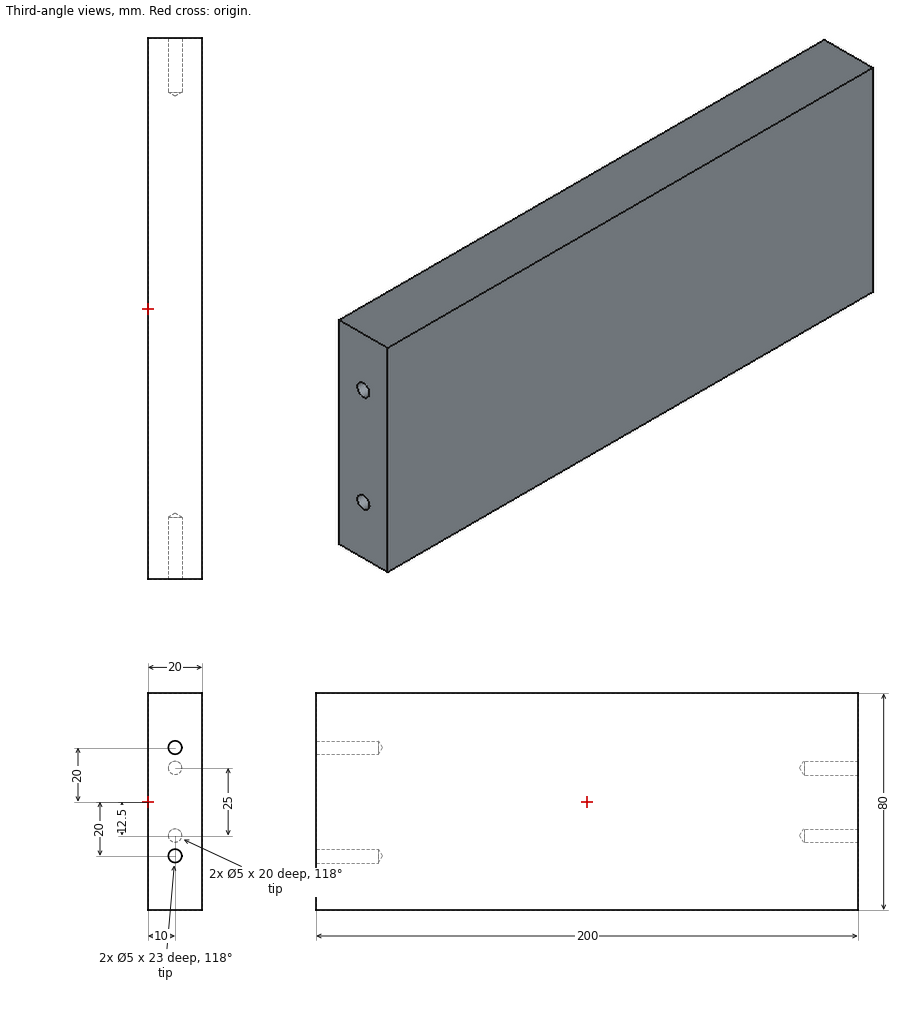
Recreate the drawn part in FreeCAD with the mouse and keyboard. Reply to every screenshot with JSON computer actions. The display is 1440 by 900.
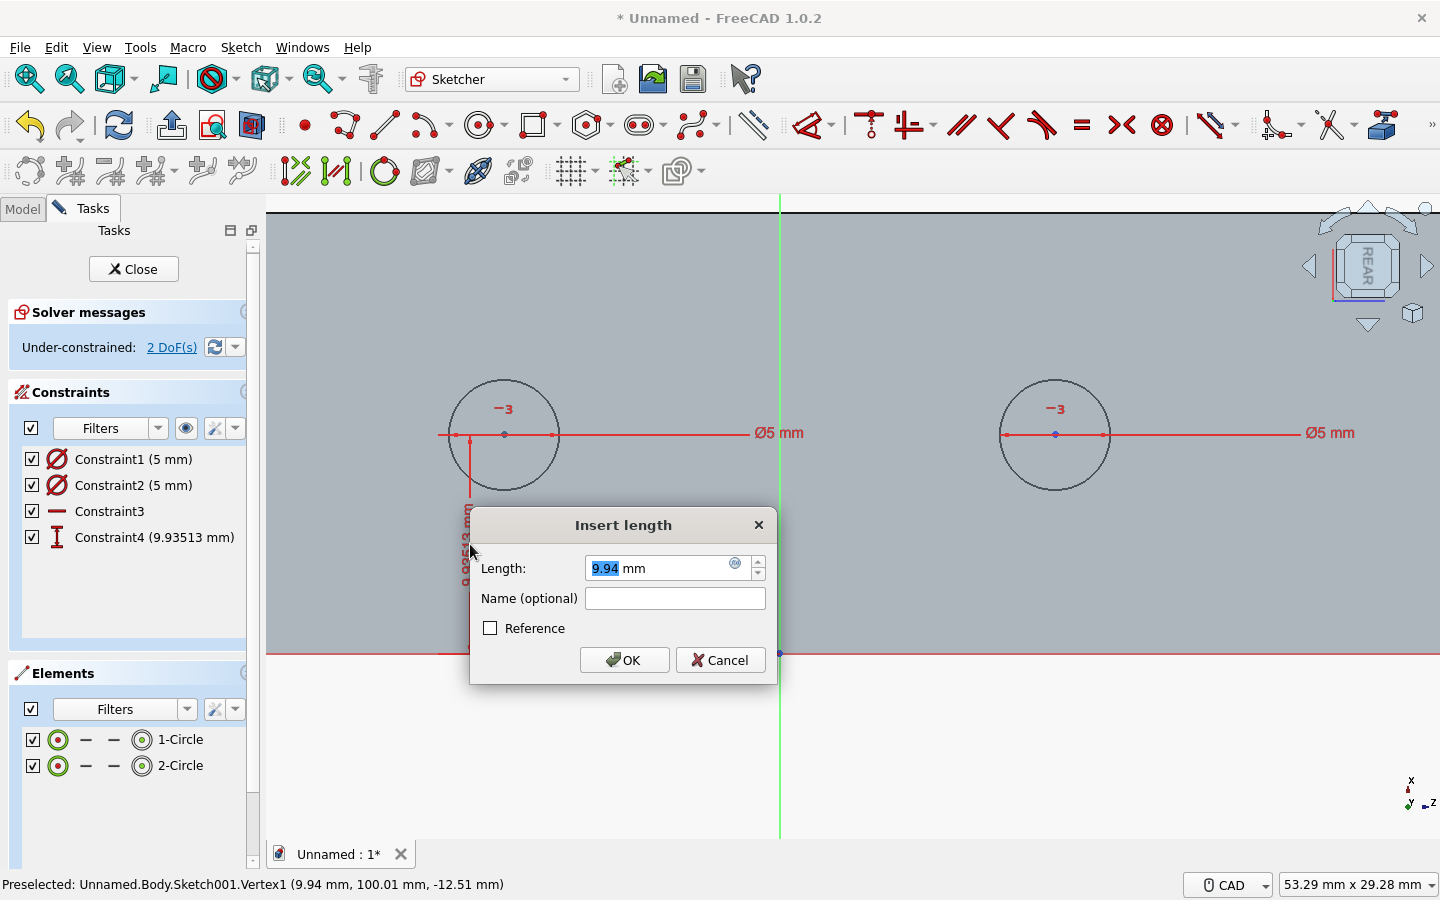
{"action": "type", "text": "10"}
{"action": "key", "text": "Return"}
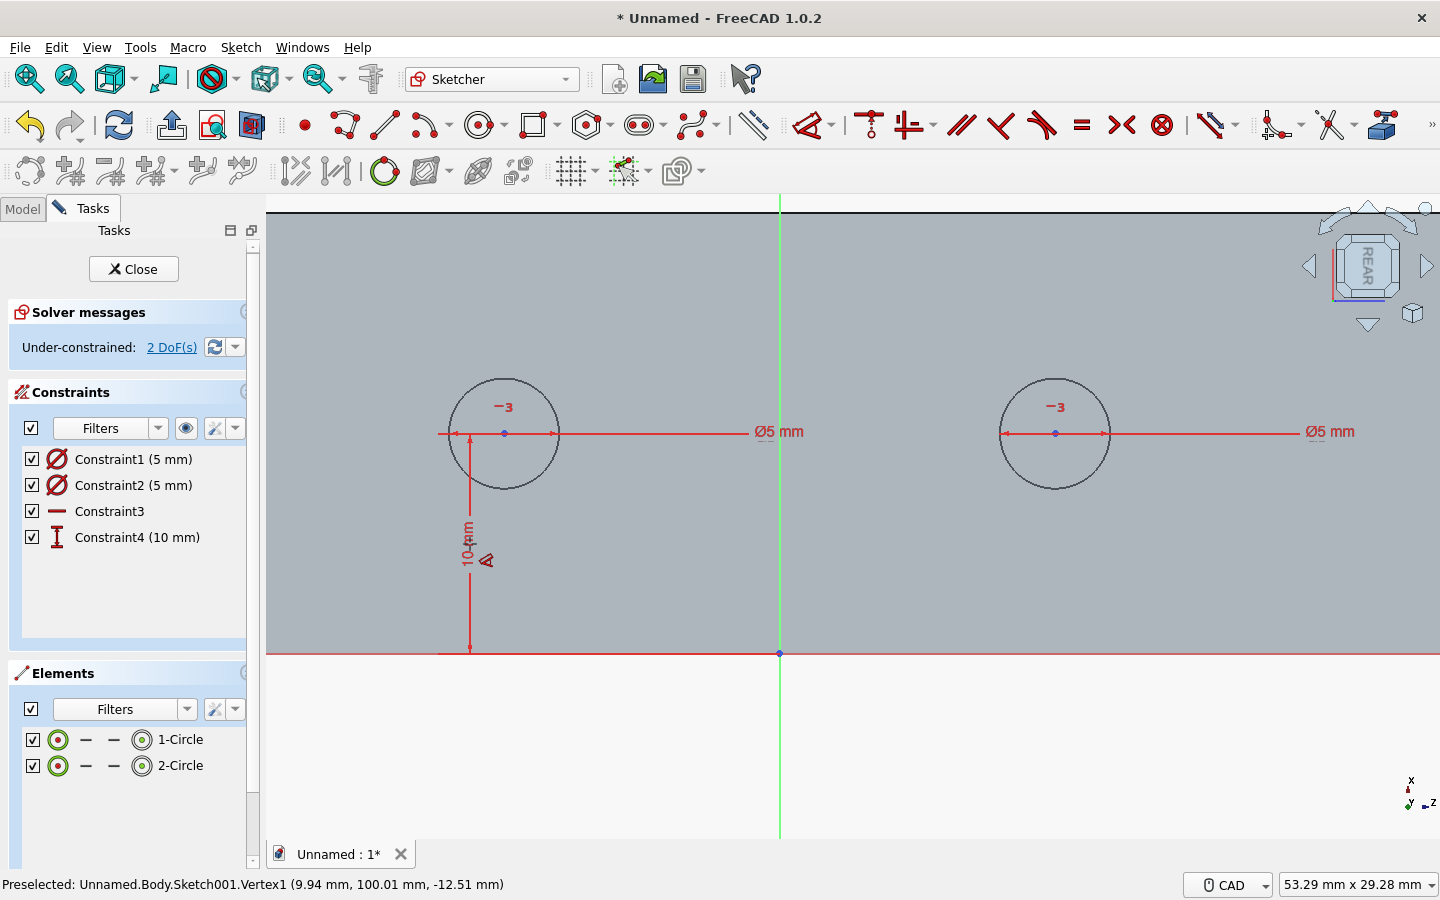
{"action": "left_click", "coordinate": [504, 434]}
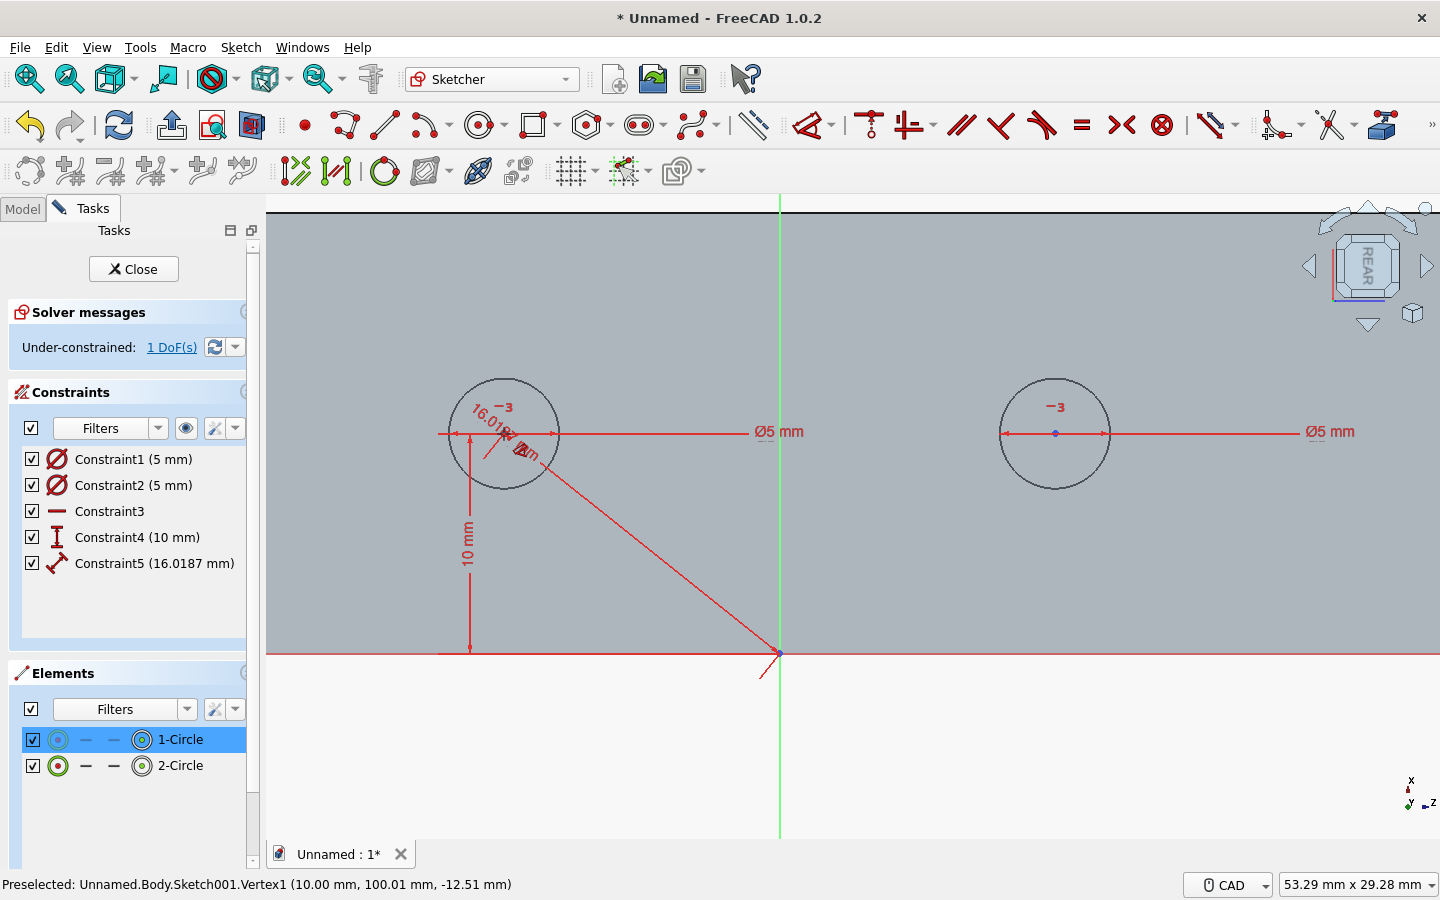
{"action": "left_click", "coordinate": [1055, 434]}
{"action": "left_click", "coordinate": [653, 400]}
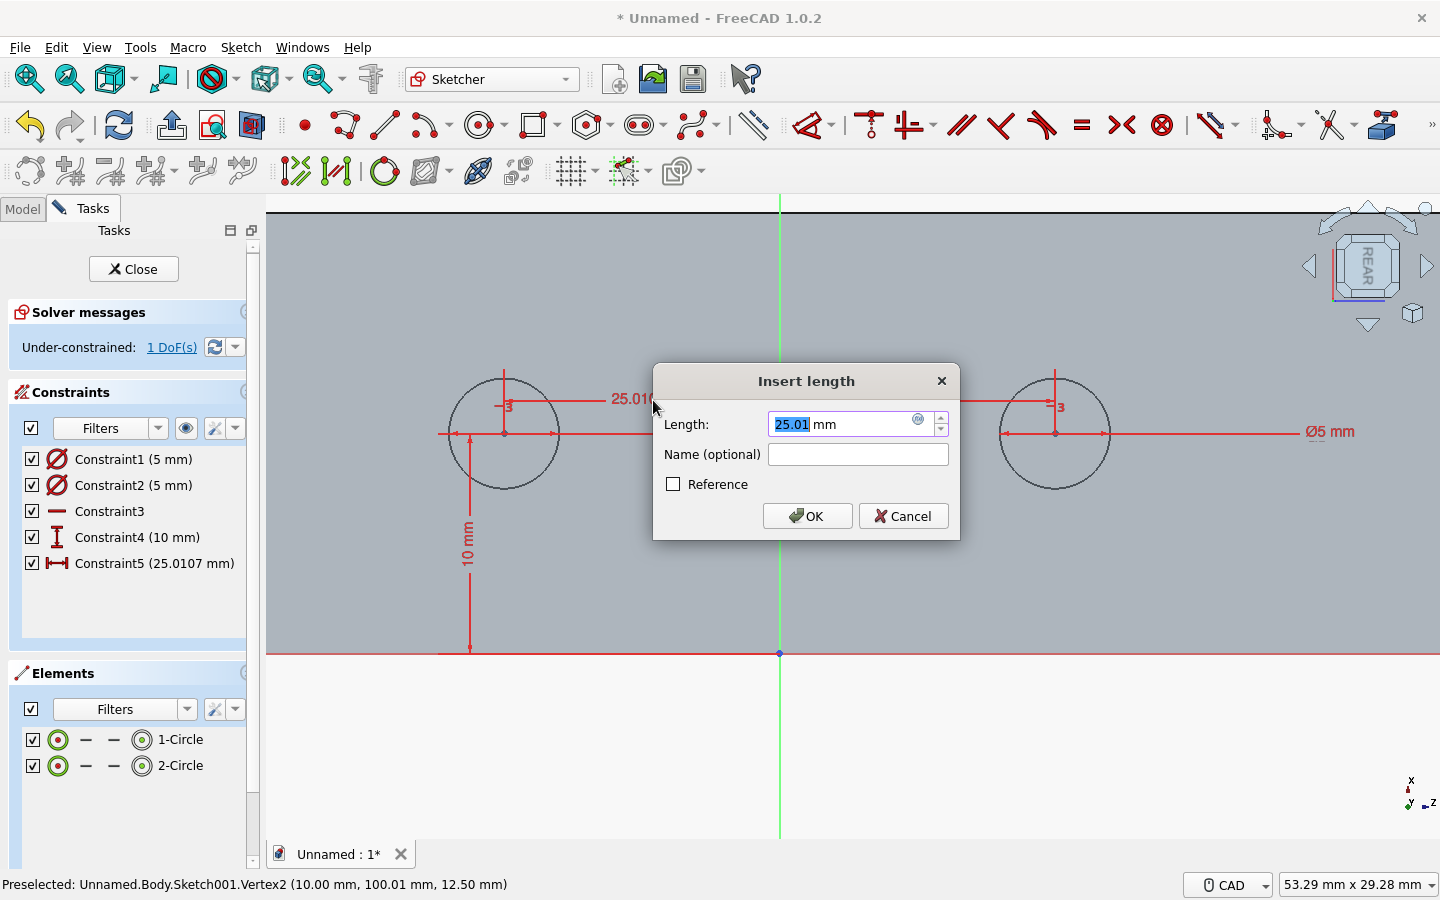
{"action": "type", "text": "25"}
{"action": "key", "text": "Return"}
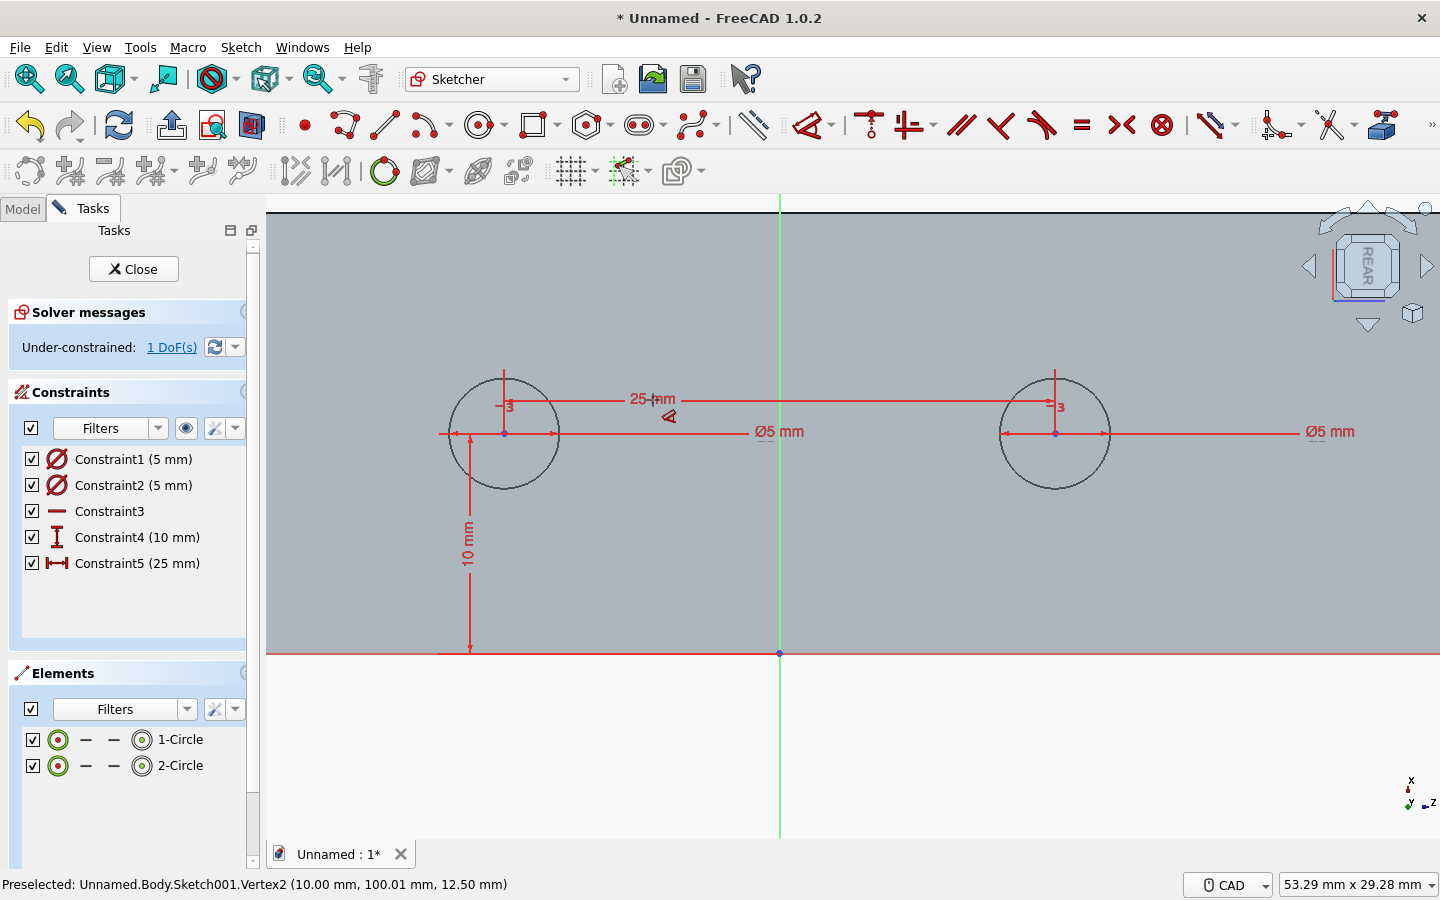
{"action": "left_click", "coordinate": [504, 434]}
{"action": "left_click", "coordinate": [642, 688]}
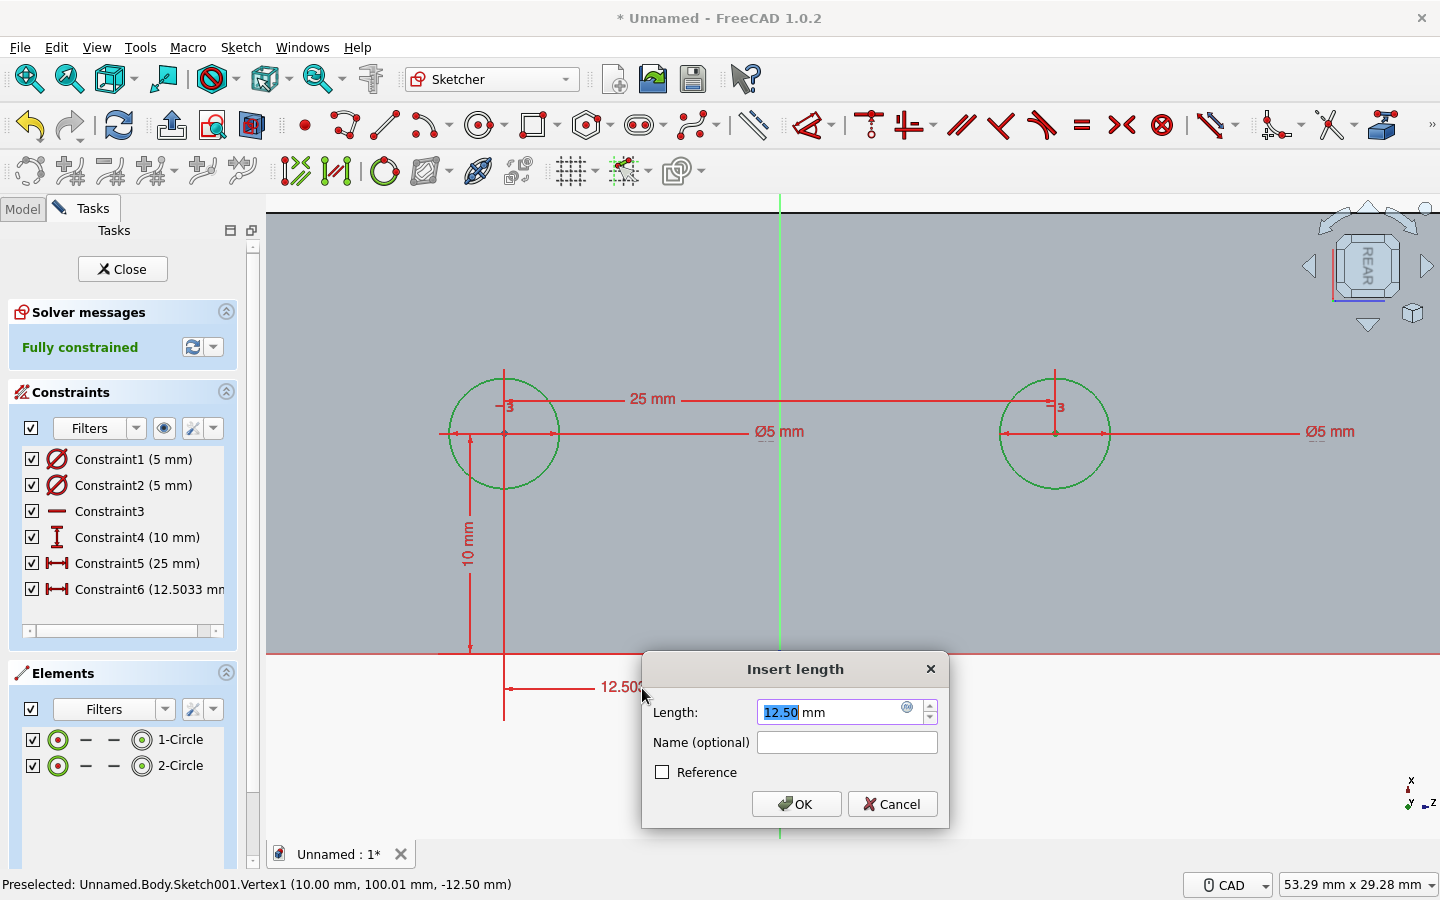
{"action": "type", "text": "12.5"}
{"action": "key", "text": "Return"}
{"action": "key", "text": "Escape"}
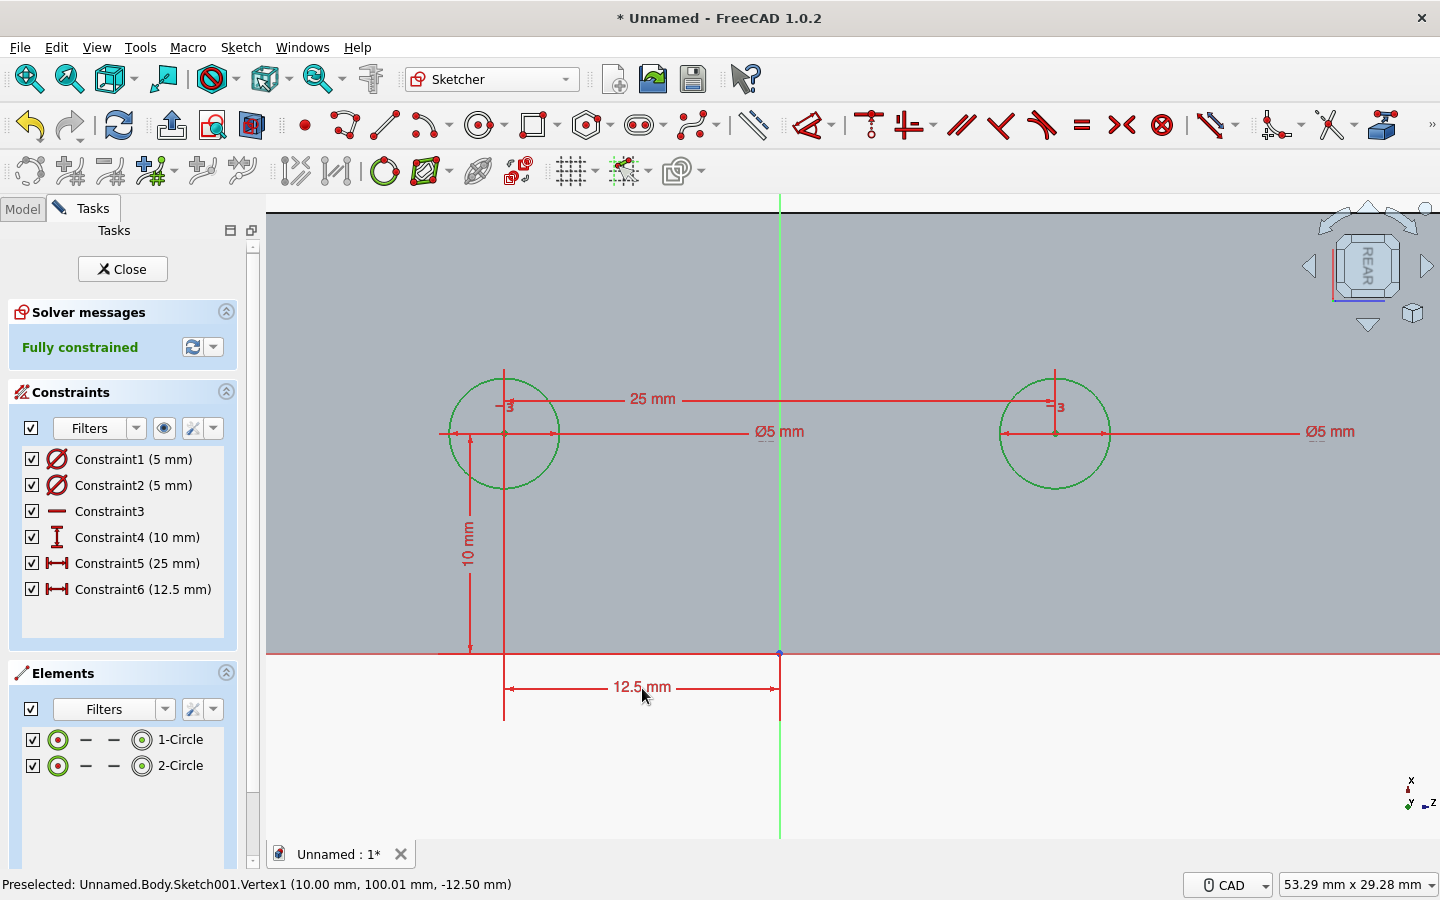
{"action": "left_click", "coordinate": [123, 269]}